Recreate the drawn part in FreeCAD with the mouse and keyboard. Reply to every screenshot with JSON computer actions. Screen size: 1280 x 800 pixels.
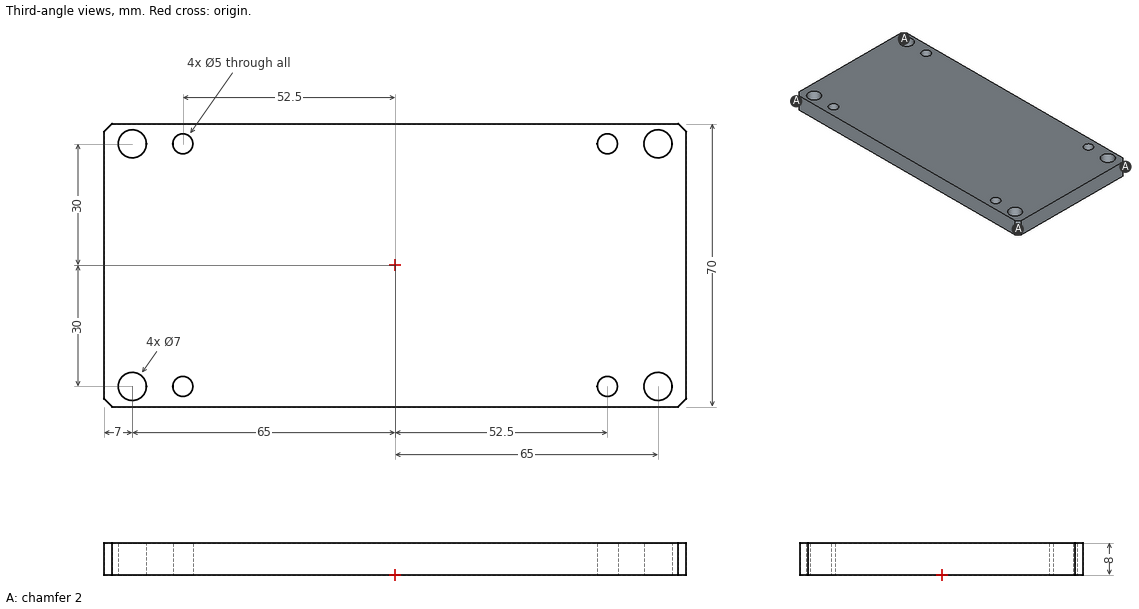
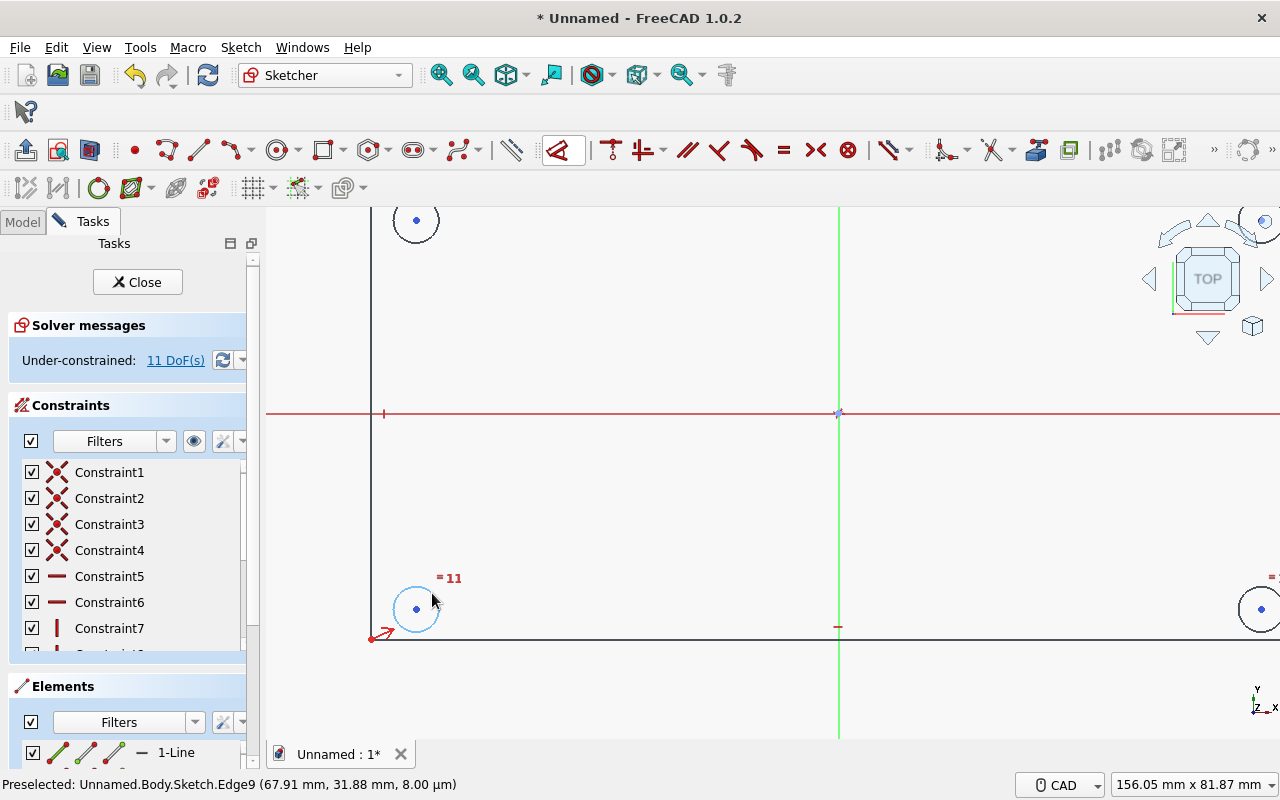
{"action": "left_click", "coordinate": [432, 593]}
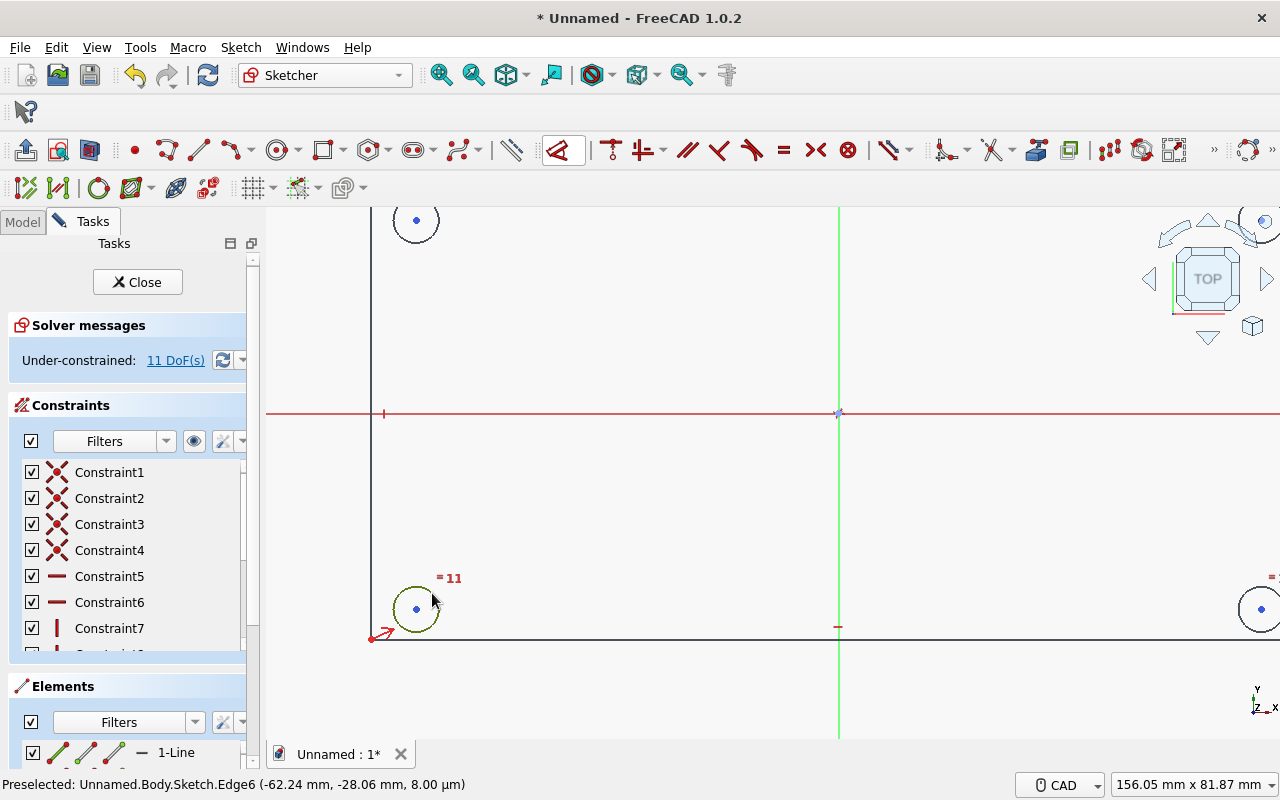
{"action": "left_click", "coordinate": [580, 150]}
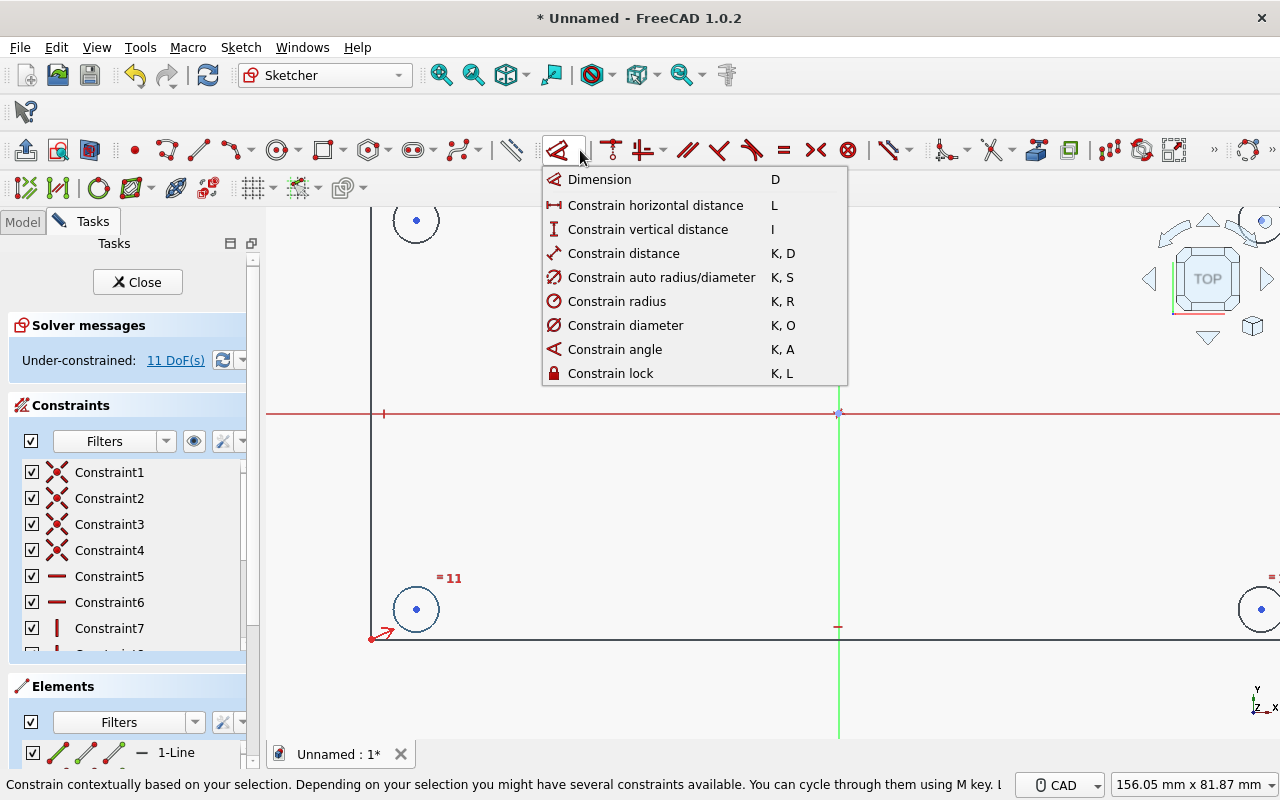
{"action": "left_click", "coordinate": [695, 325]}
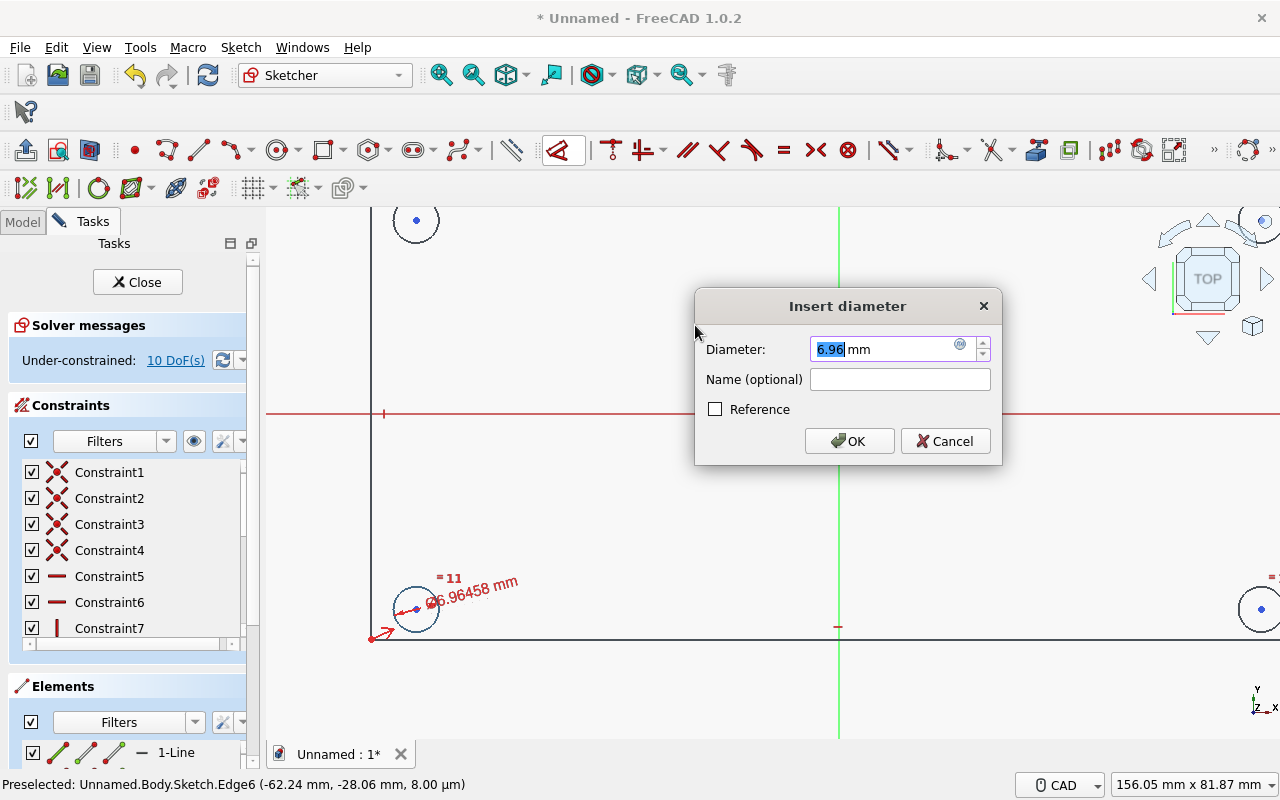
{"action": "type", "text": "7"}
{"action": "key", "text": "Return"}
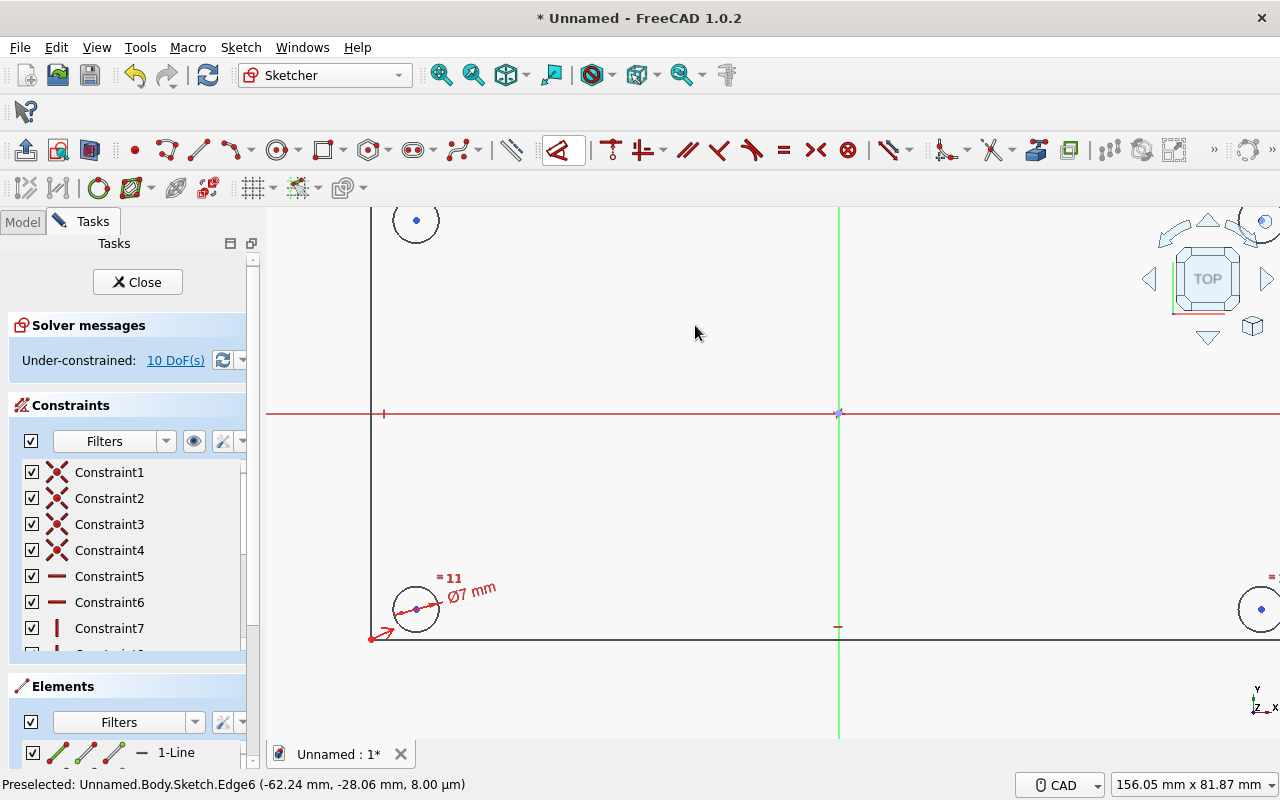
{"action": "scroll", "coordinate": [431, 593], "scroll_direction": "down", "scroll_amount": 2}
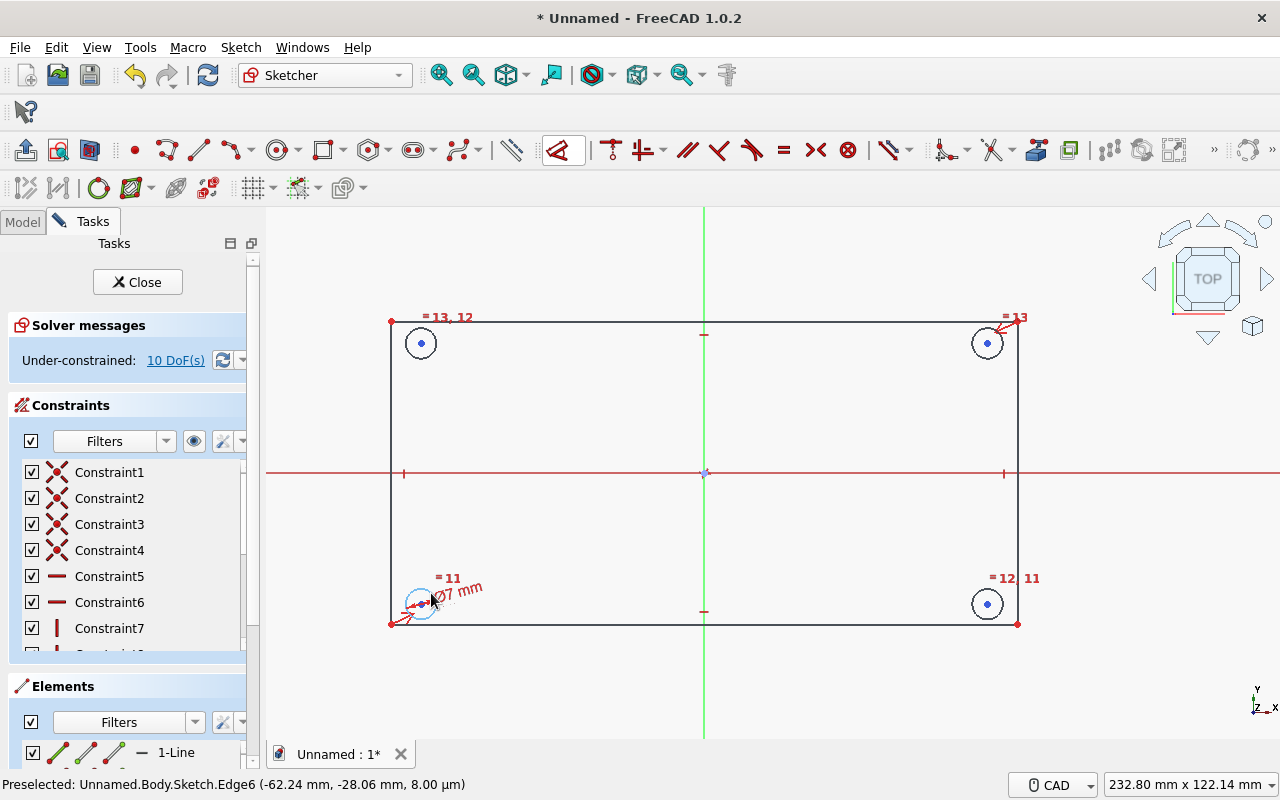
{"action": "left_click", "coordinate": [1018, 534]}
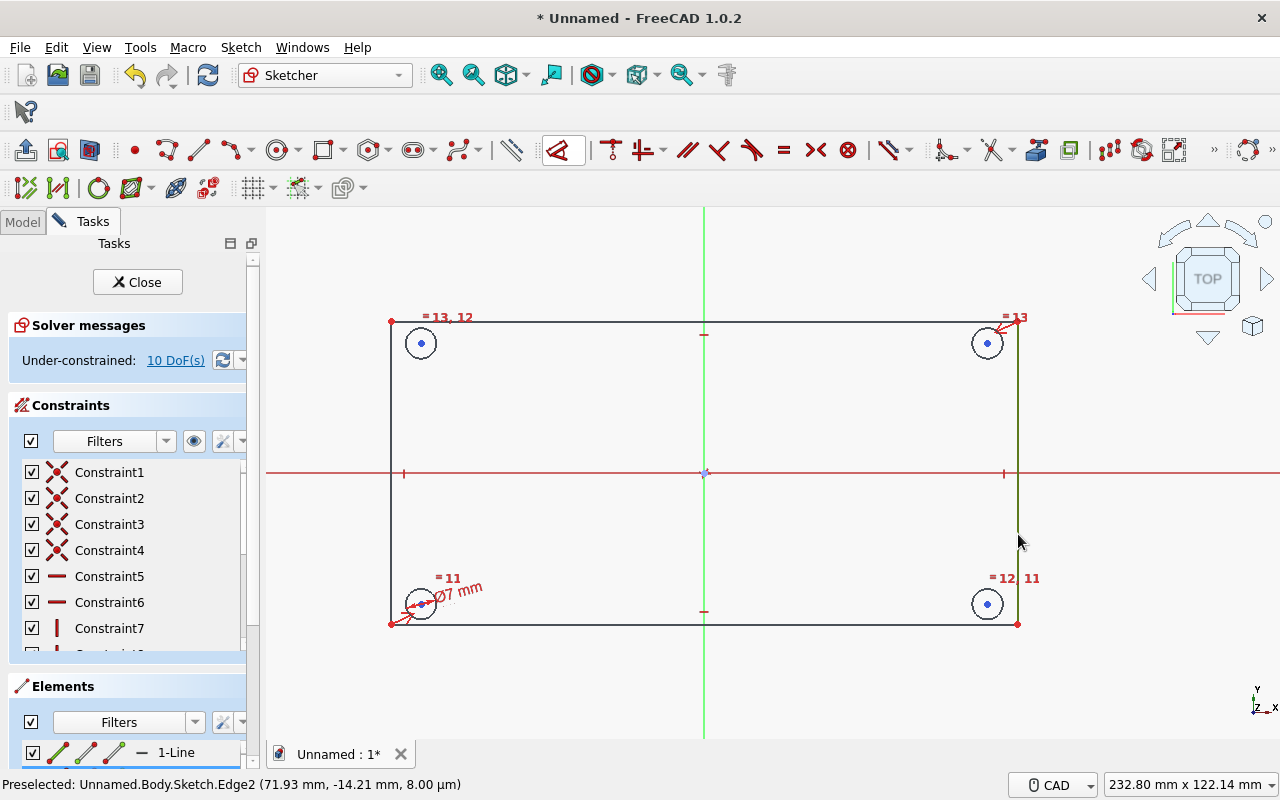
{"action": "key", "text": "i"}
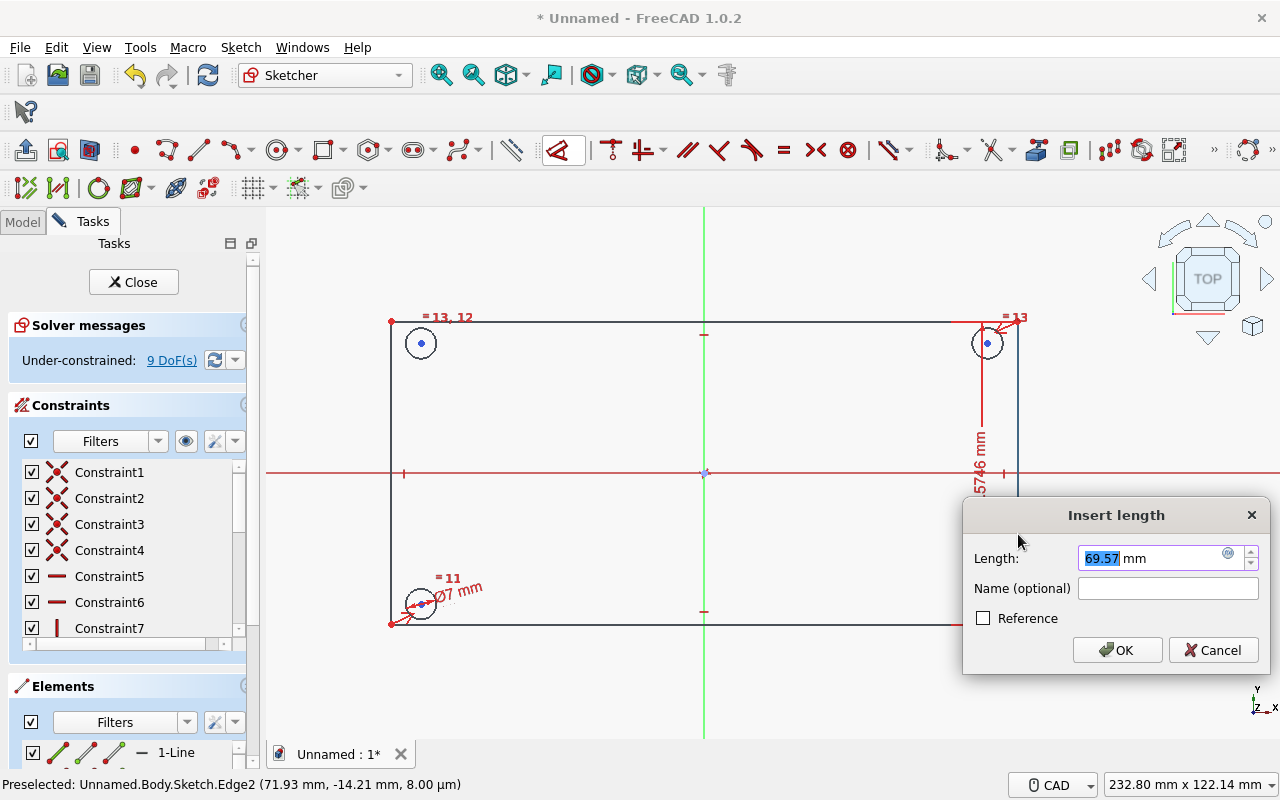
{"action": "type", "text": "70"}
{"action": "key", "text": "Return"}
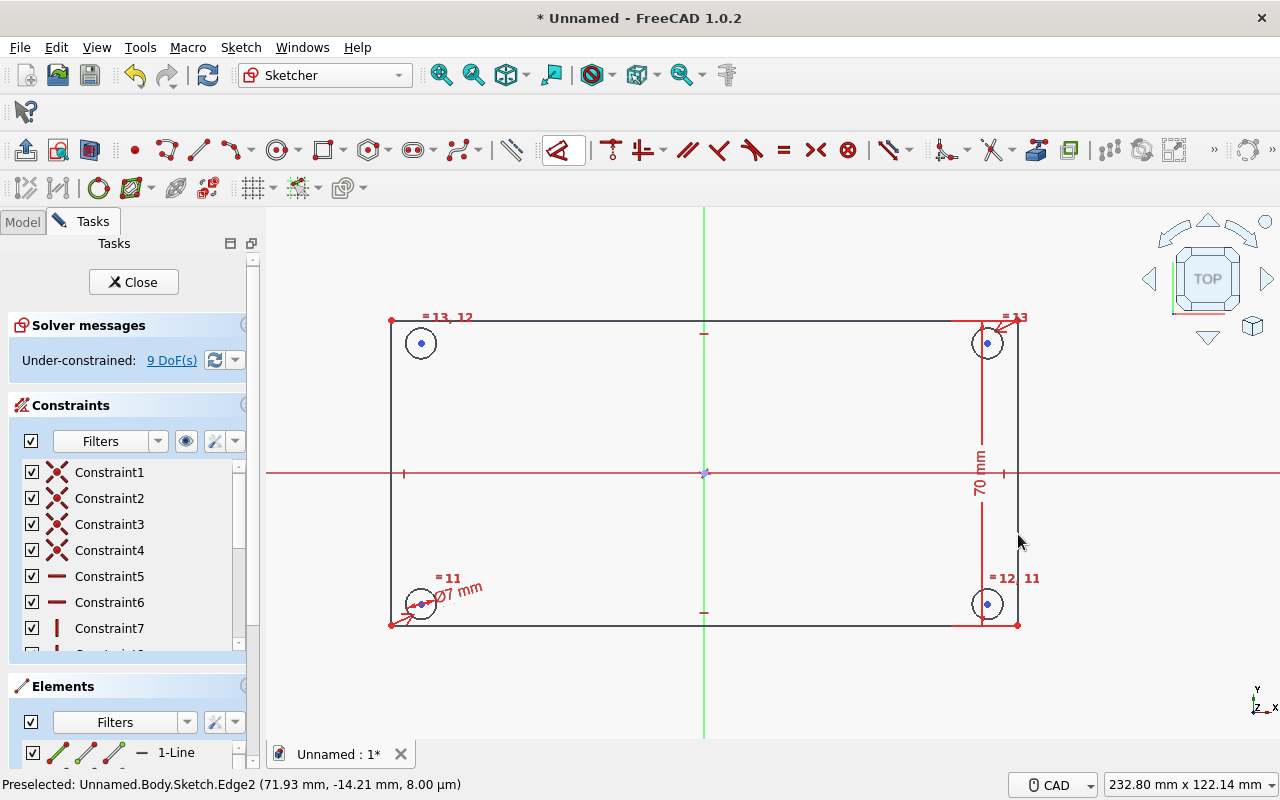
{"action": "left_click", "coordinate": [421, 604]}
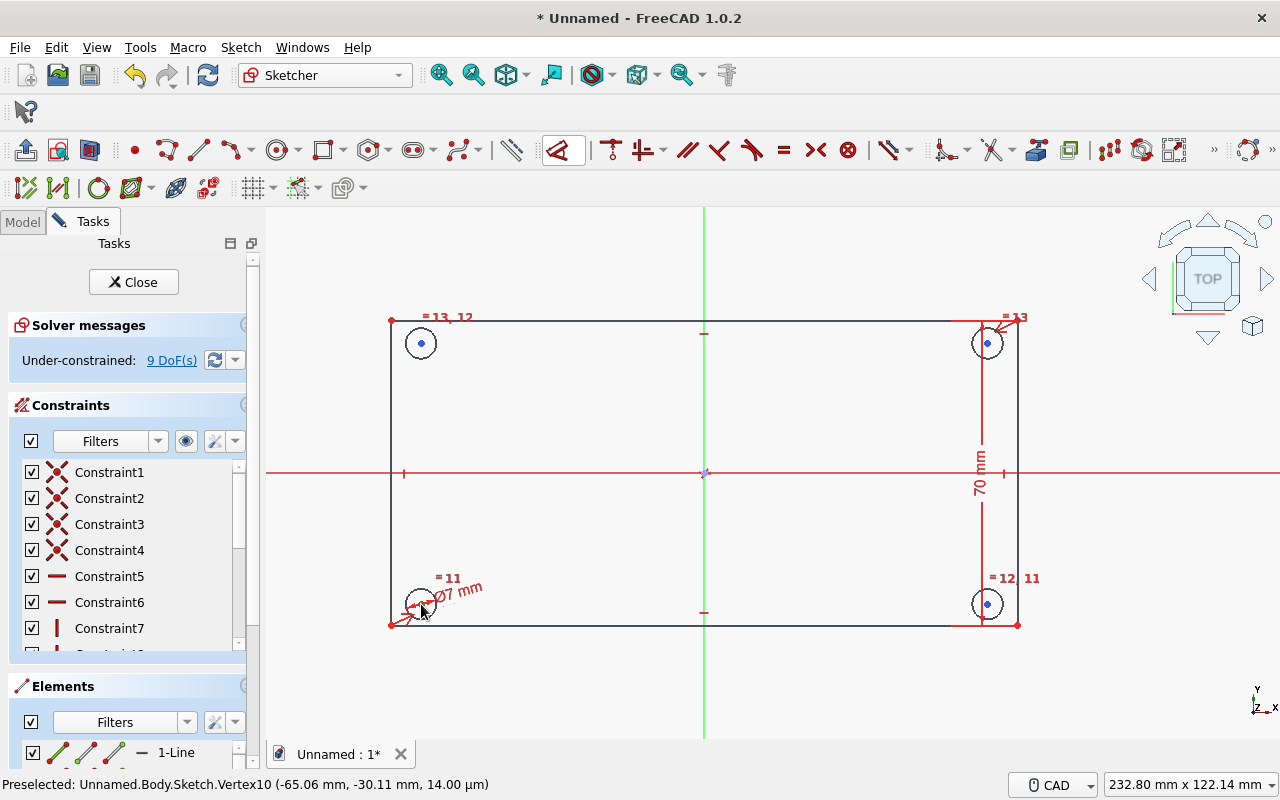
{"action": "left_click", "coordinate": [580, 150]}